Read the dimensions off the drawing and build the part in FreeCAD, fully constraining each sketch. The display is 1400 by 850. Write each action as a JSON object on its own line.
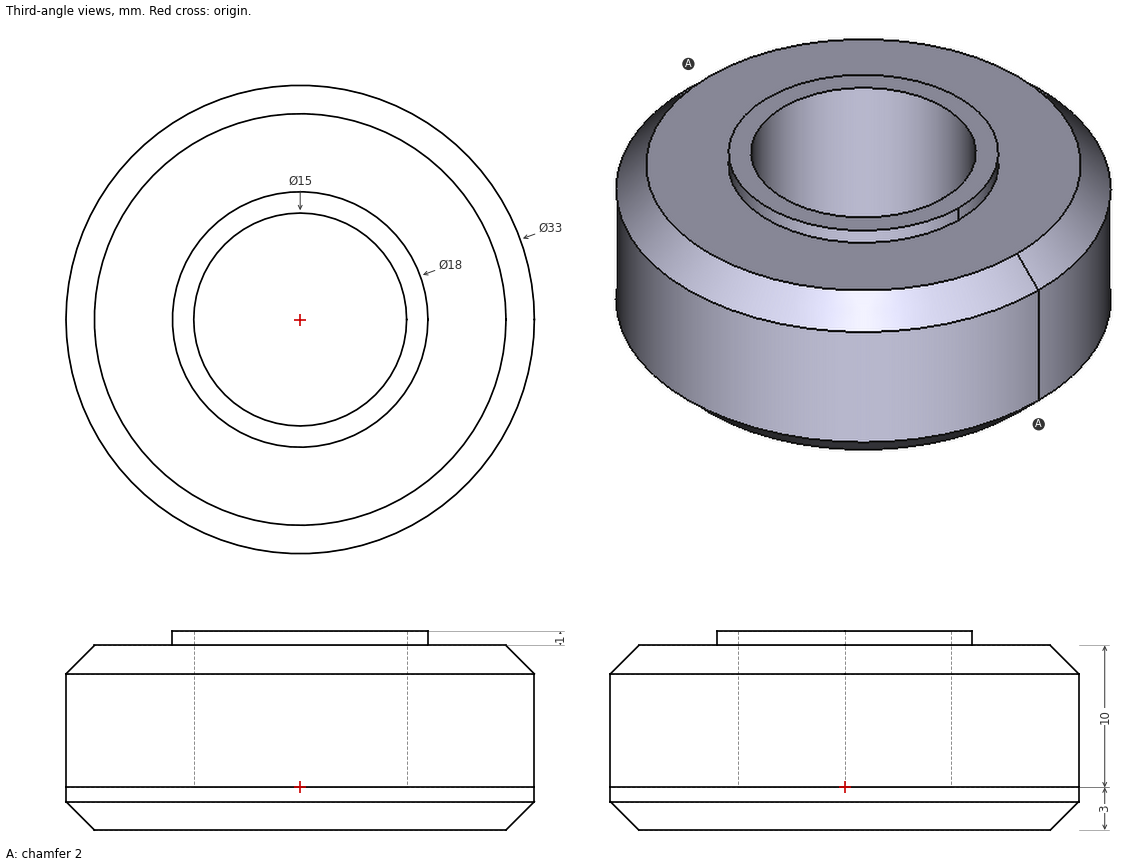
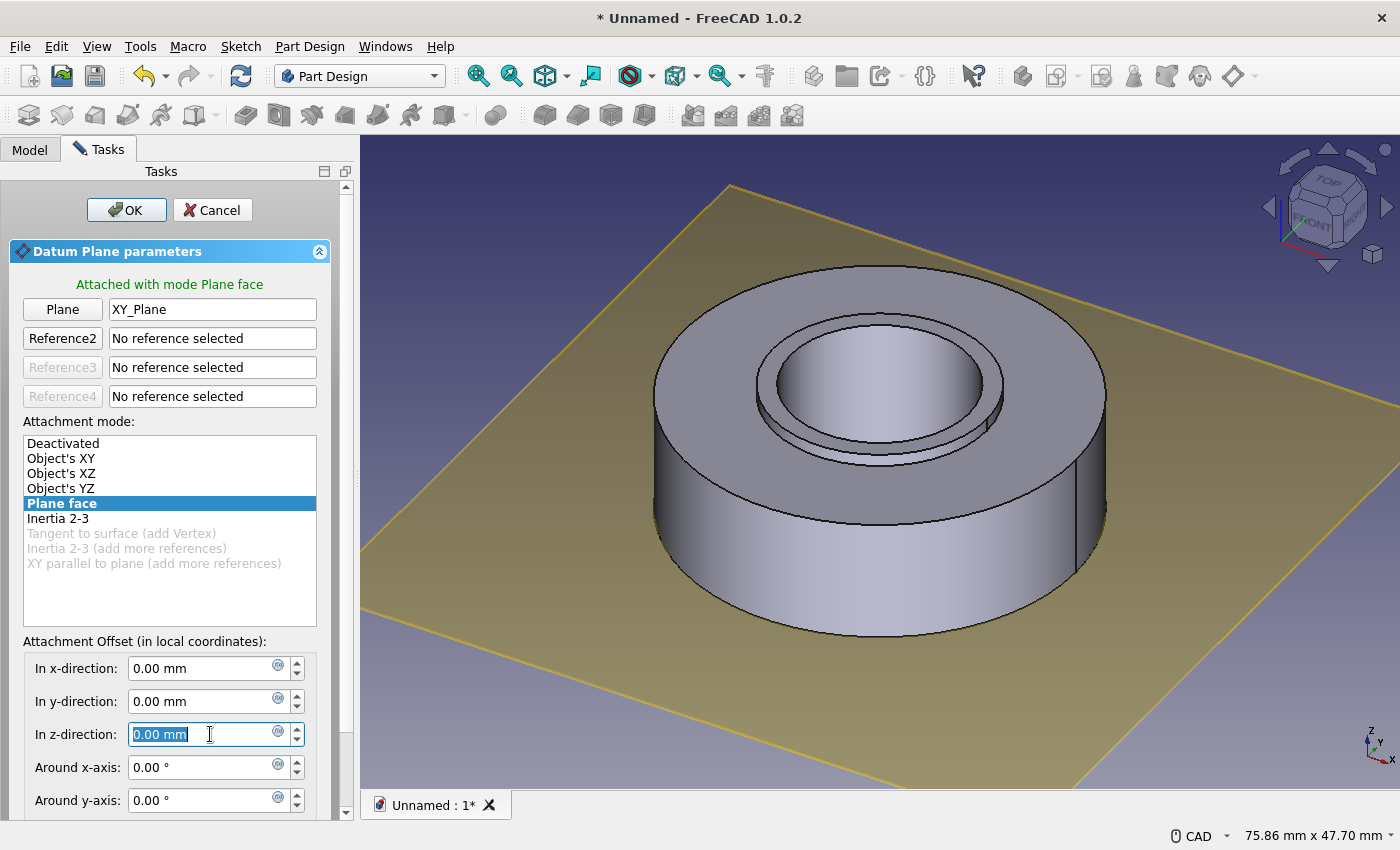
{"action": "type", "text": "-3"}
{"action": "key", "text": "Tab"}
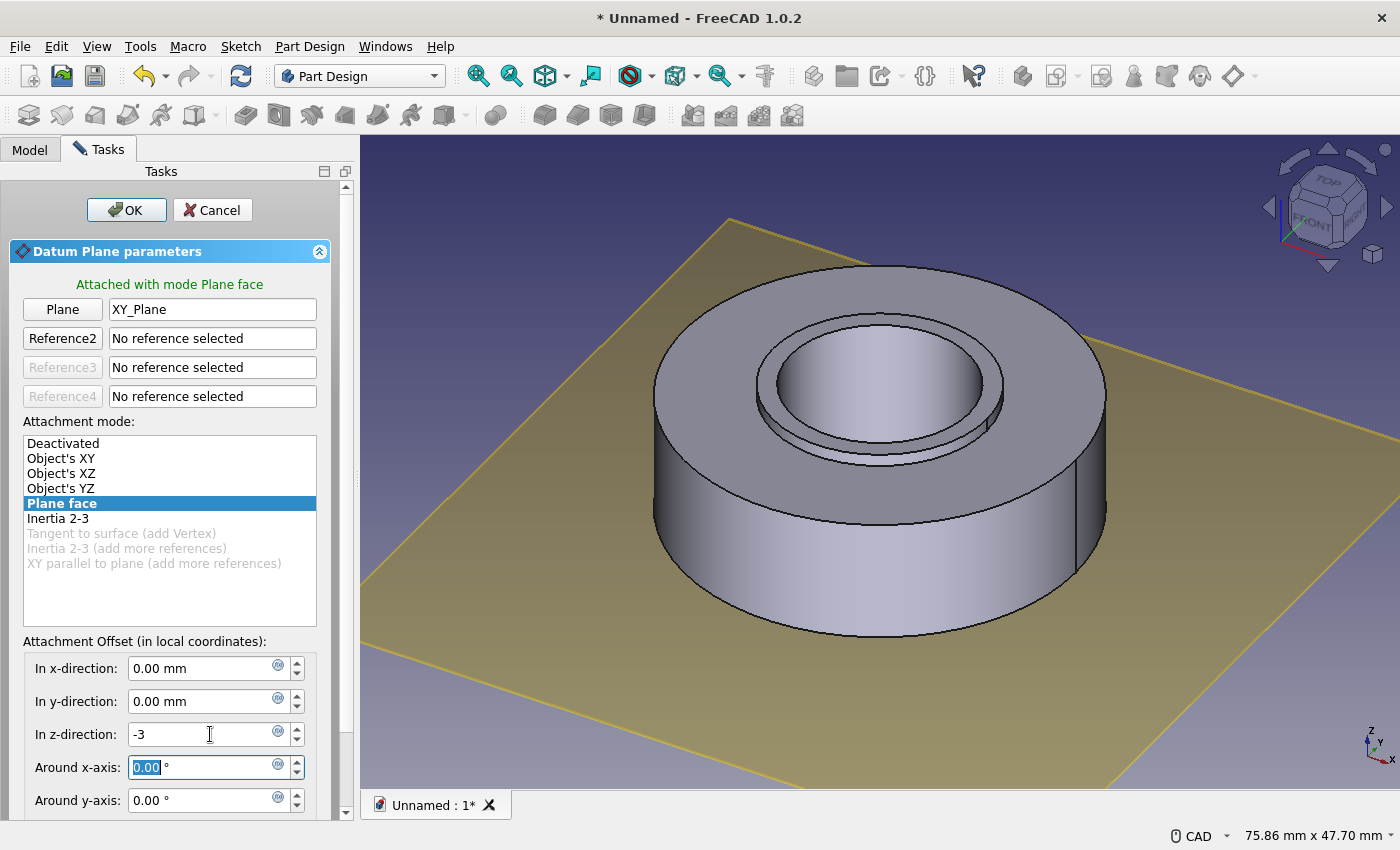
{"action": "left_click", "coordinate": [127, 210]}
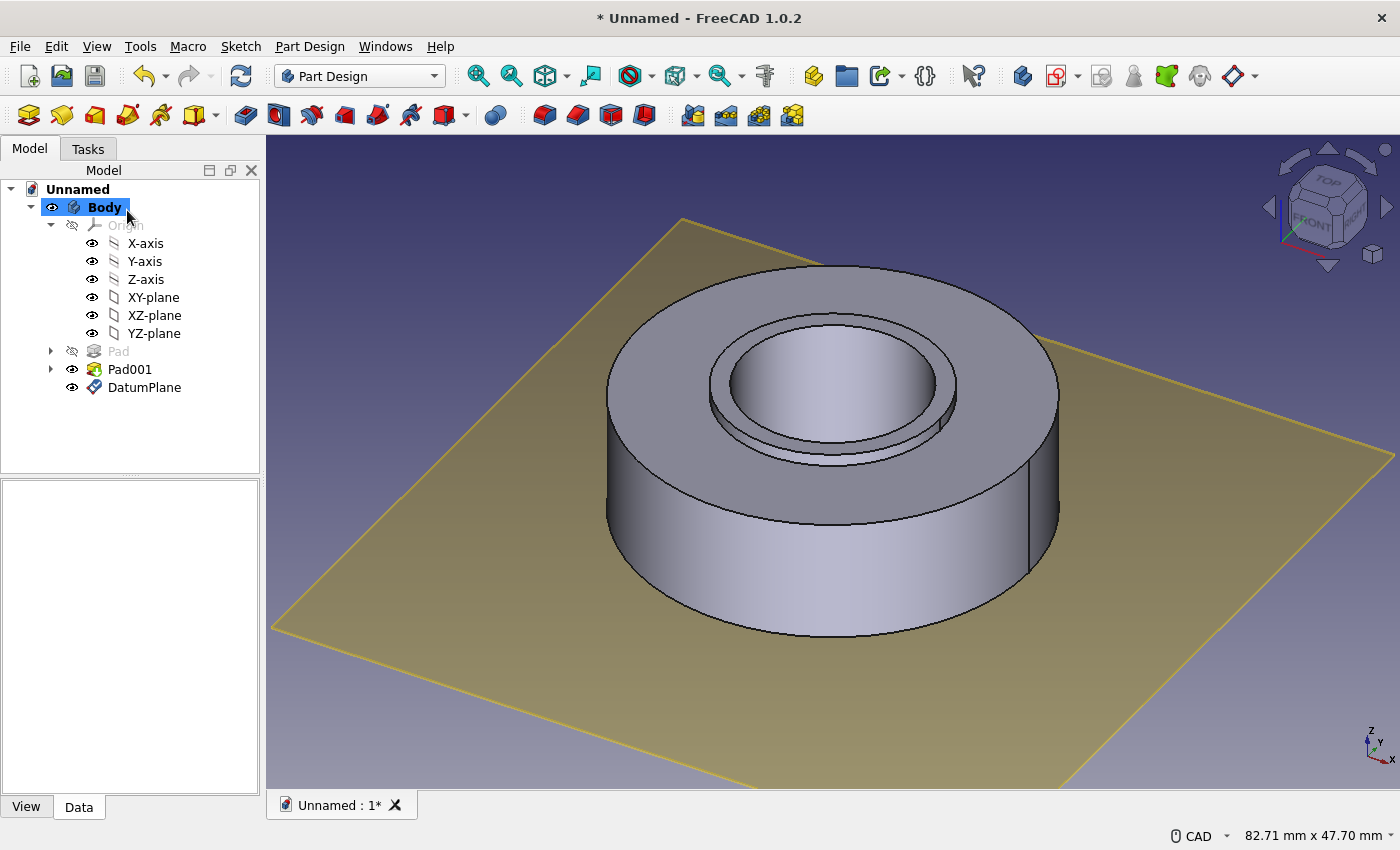
{"action": "left_click", "coordinate": [117, 387]}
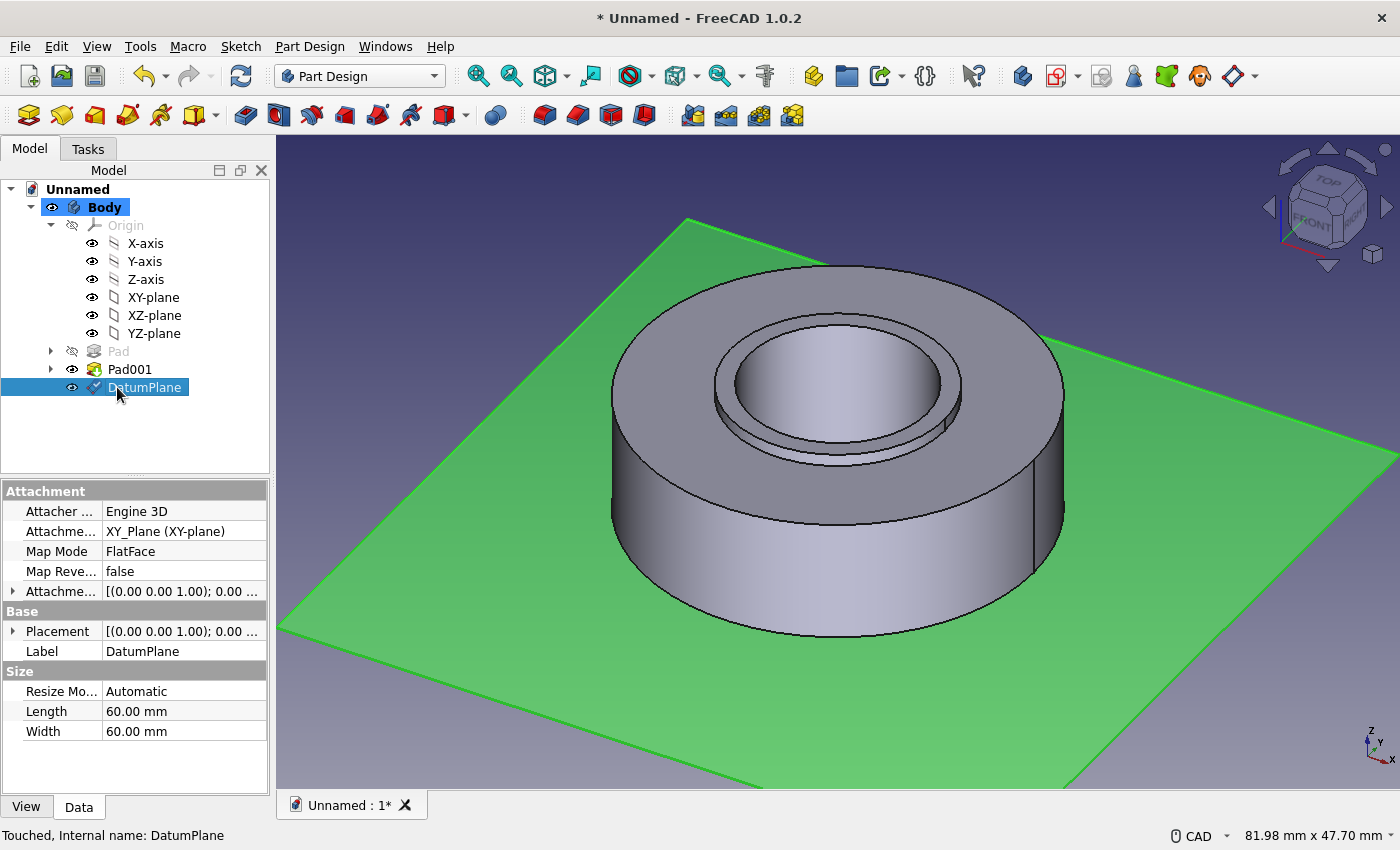
{"action": "left_click", "coordinate": [1056, 76]}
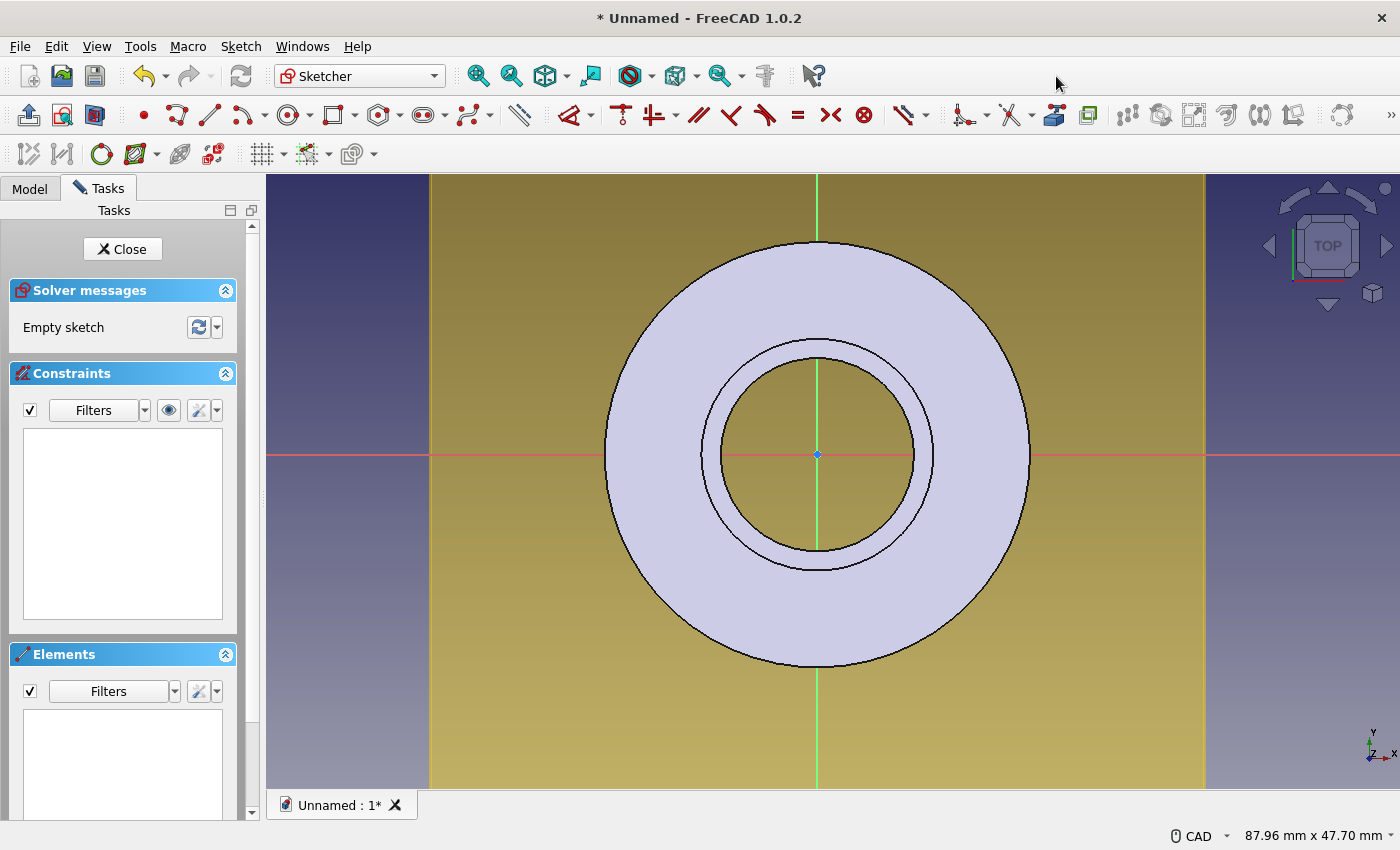
{"action": "key", "text": "q s"}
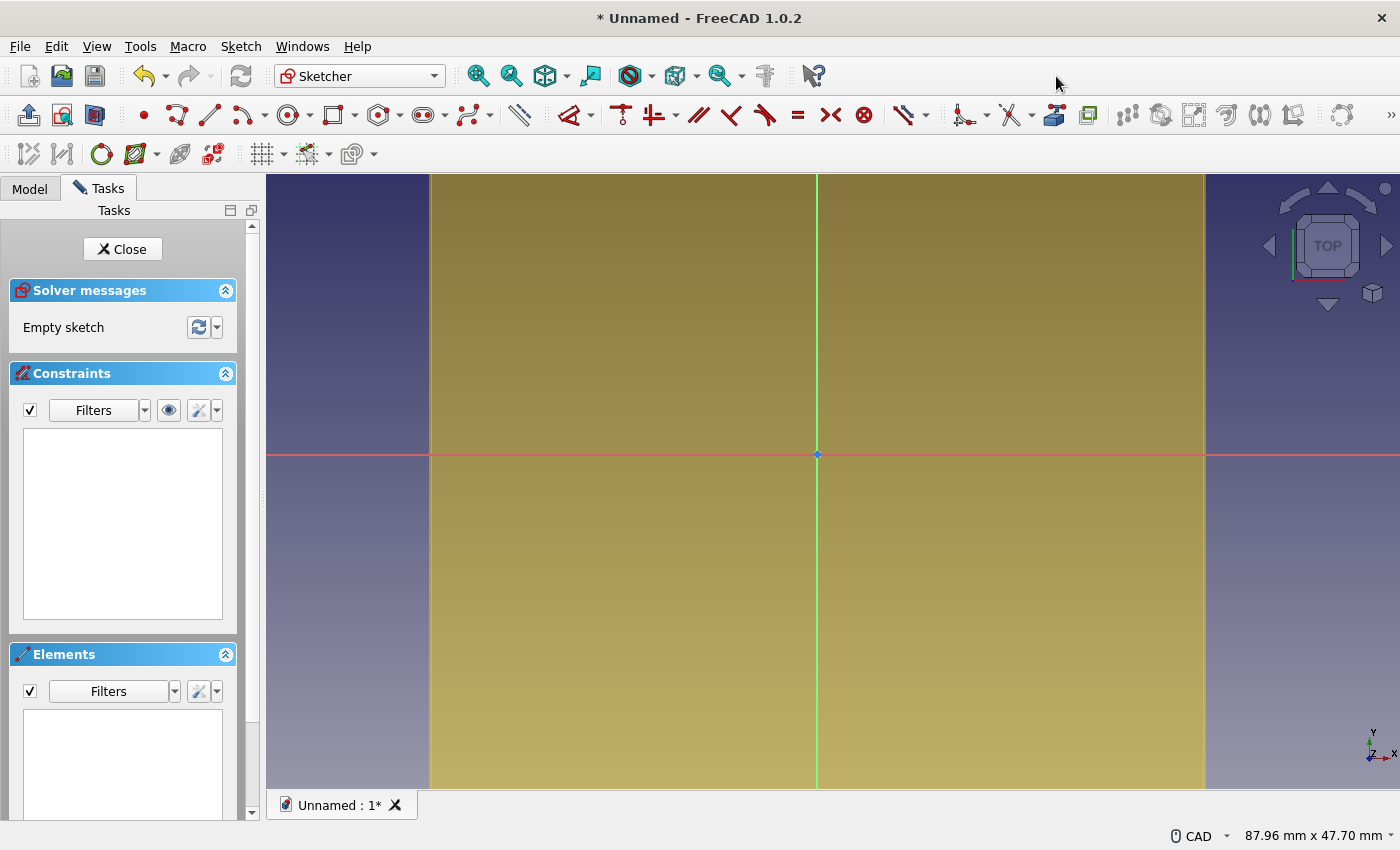
{"action": "key", "text": "g c"}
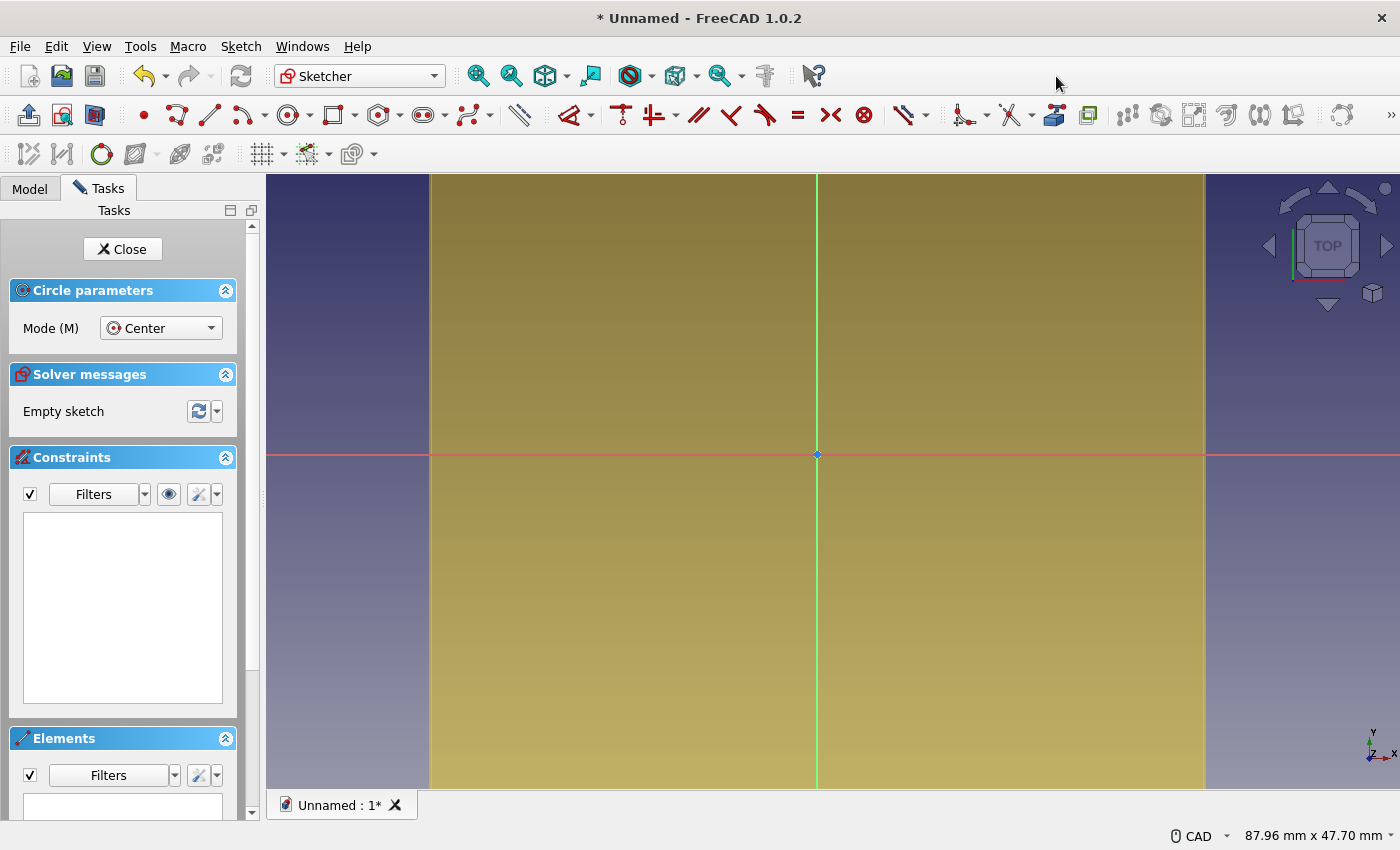
{"action": "left_click", "coordinate": [817, 455]}
{"action": "mouse_move", "coordinate": [968, 304]}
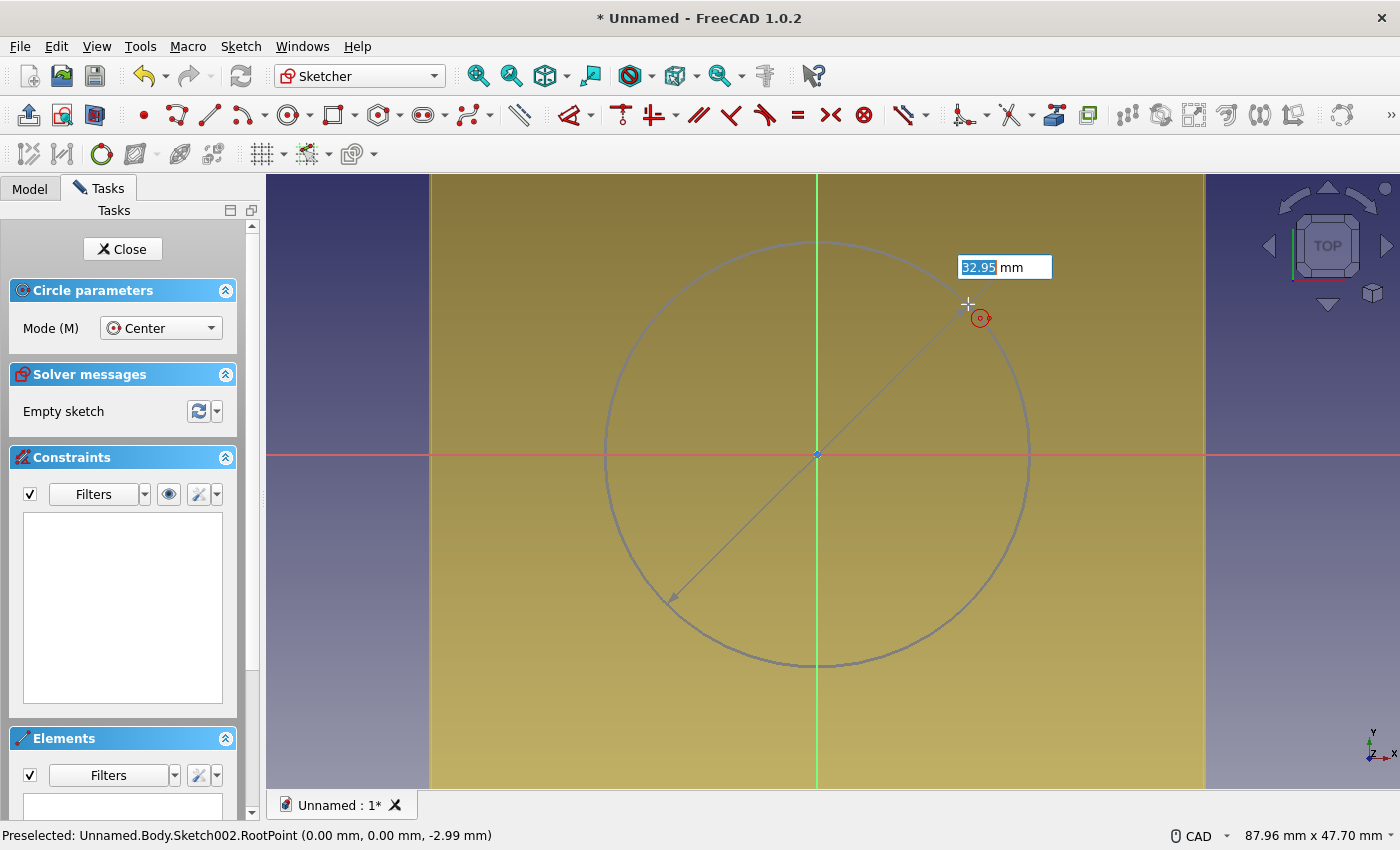
{"action": "type", "text": "33"}
{"action": "key", "text": "Return"}
{"action": "key", "text": "Escape"}